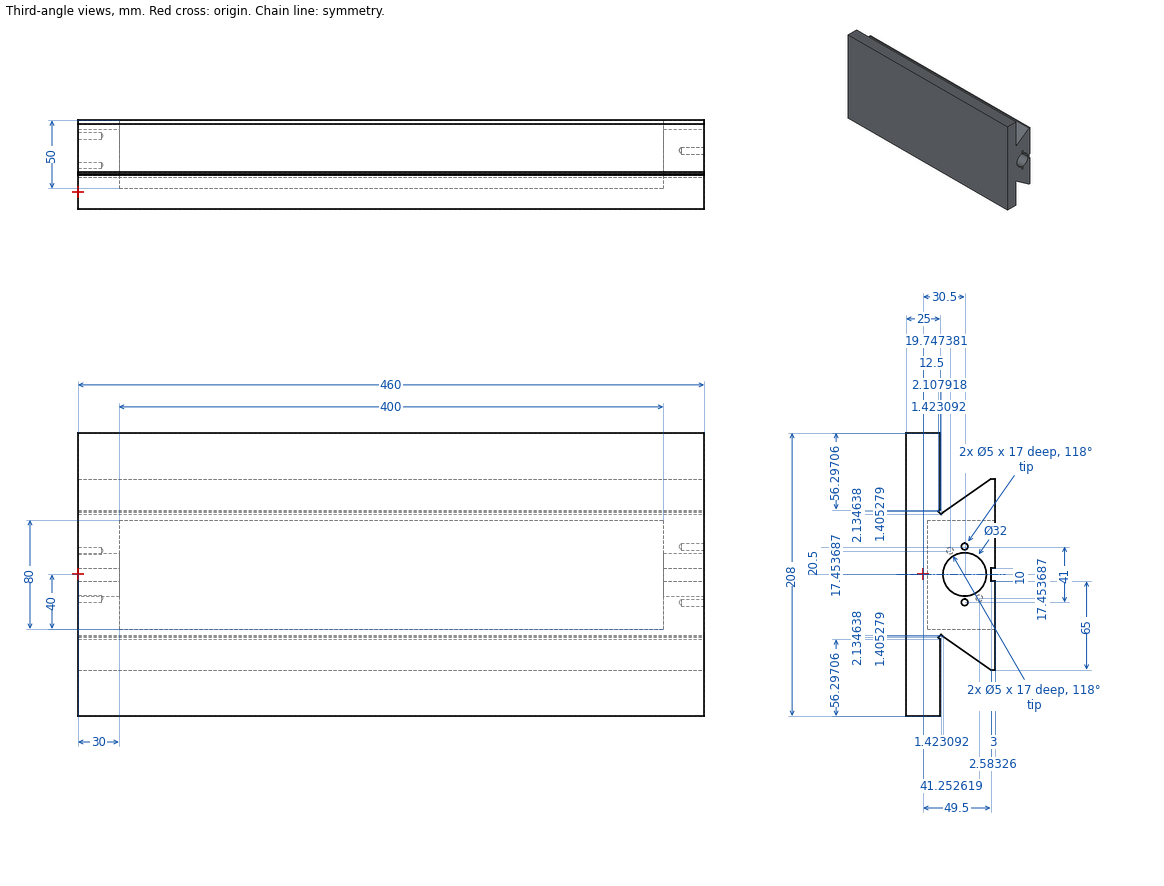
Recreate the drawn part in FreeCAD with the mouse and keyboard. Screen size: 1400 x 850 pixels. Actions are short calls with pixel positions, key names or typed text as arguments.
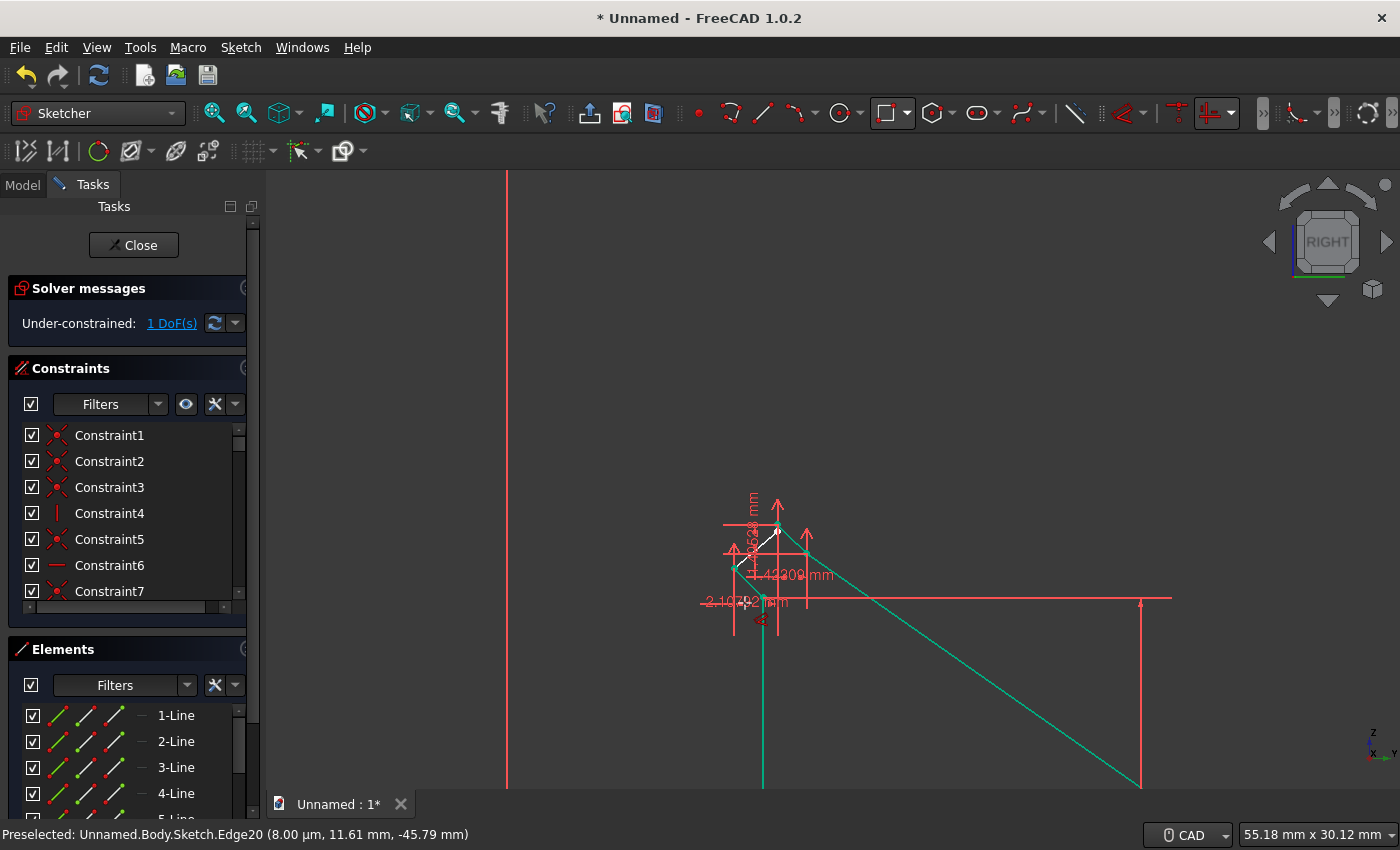
click(747, 558)
click(700, 559)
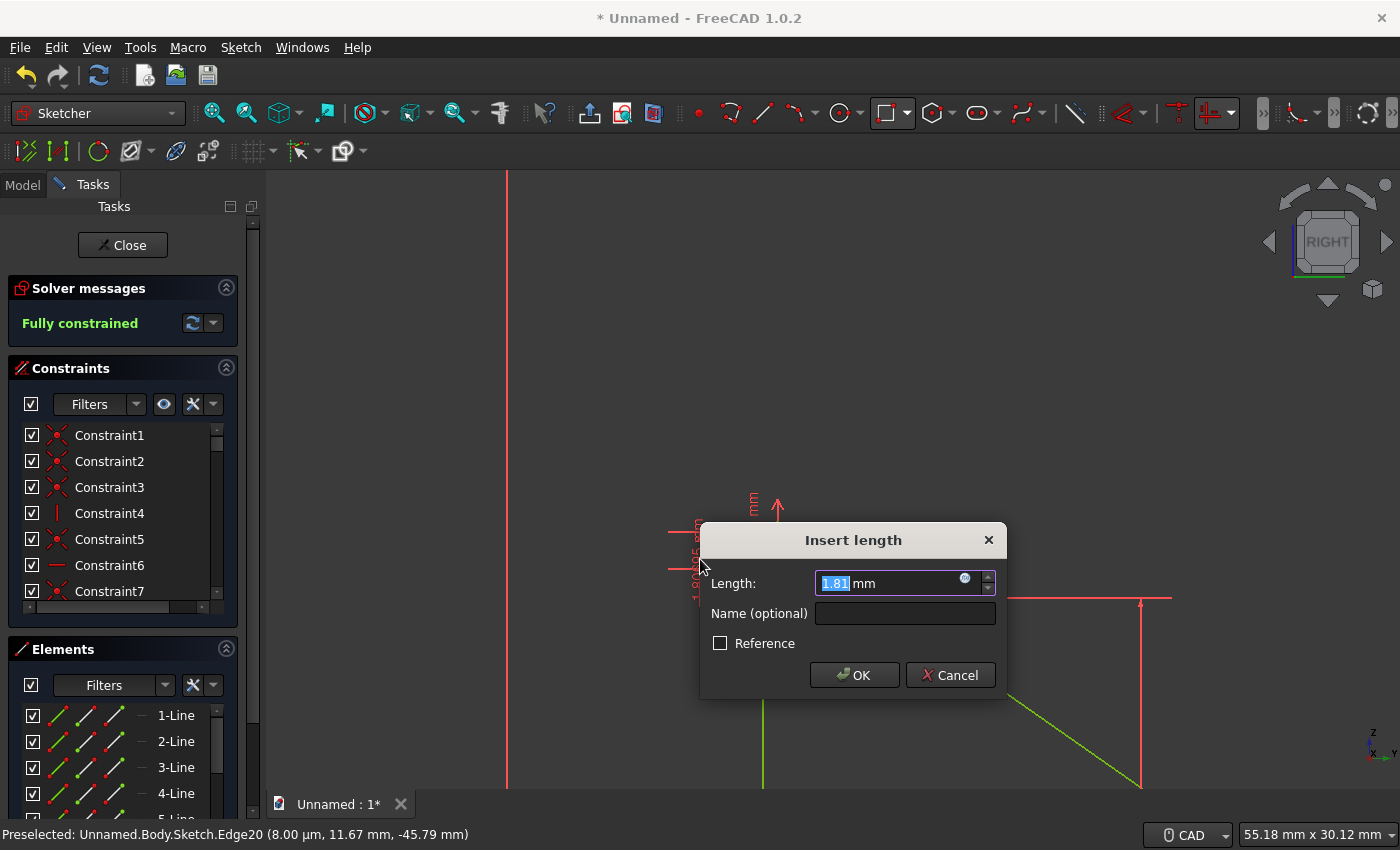
text(2.134638)
key(Return)
key(Escape)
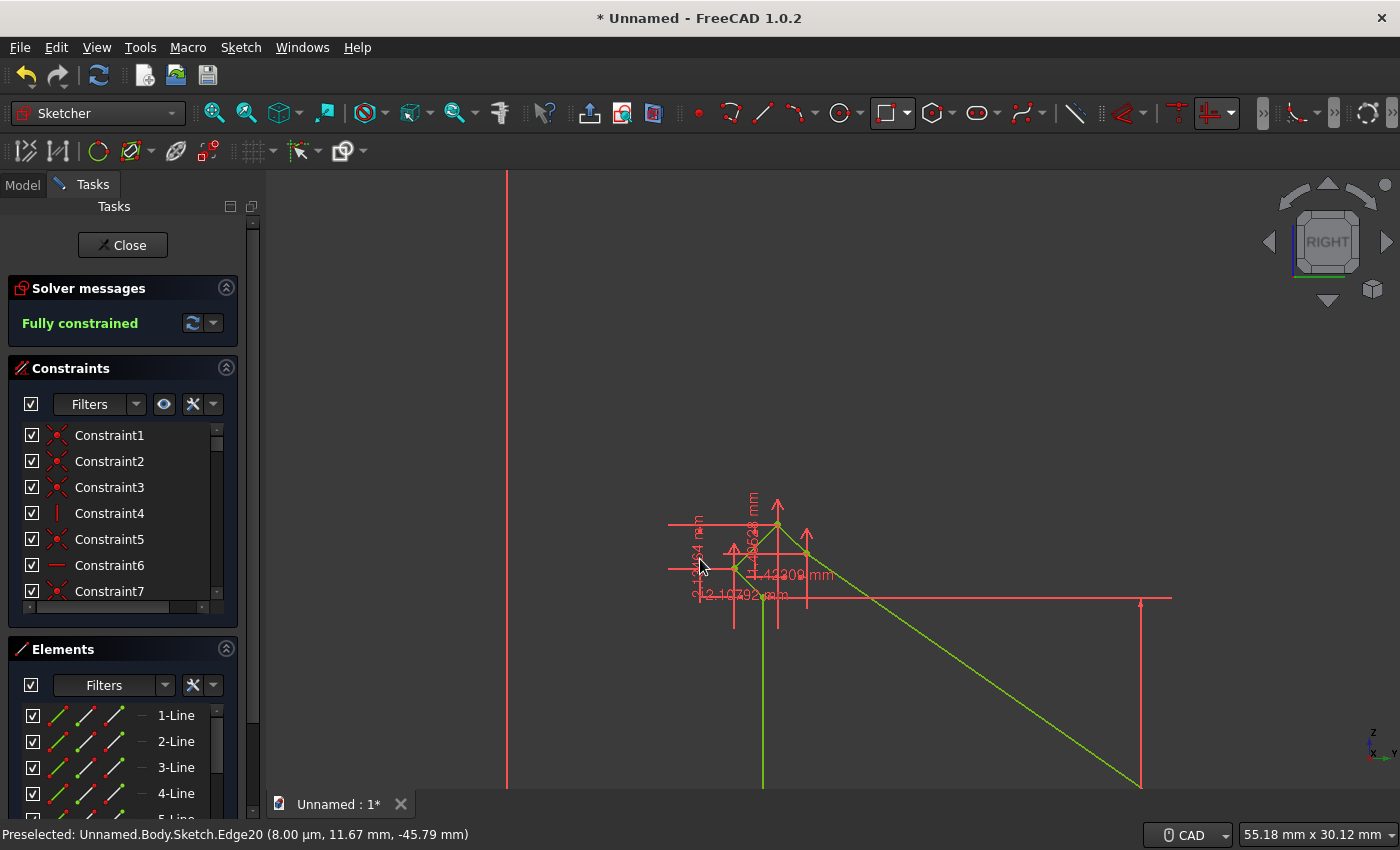
click(123, 245)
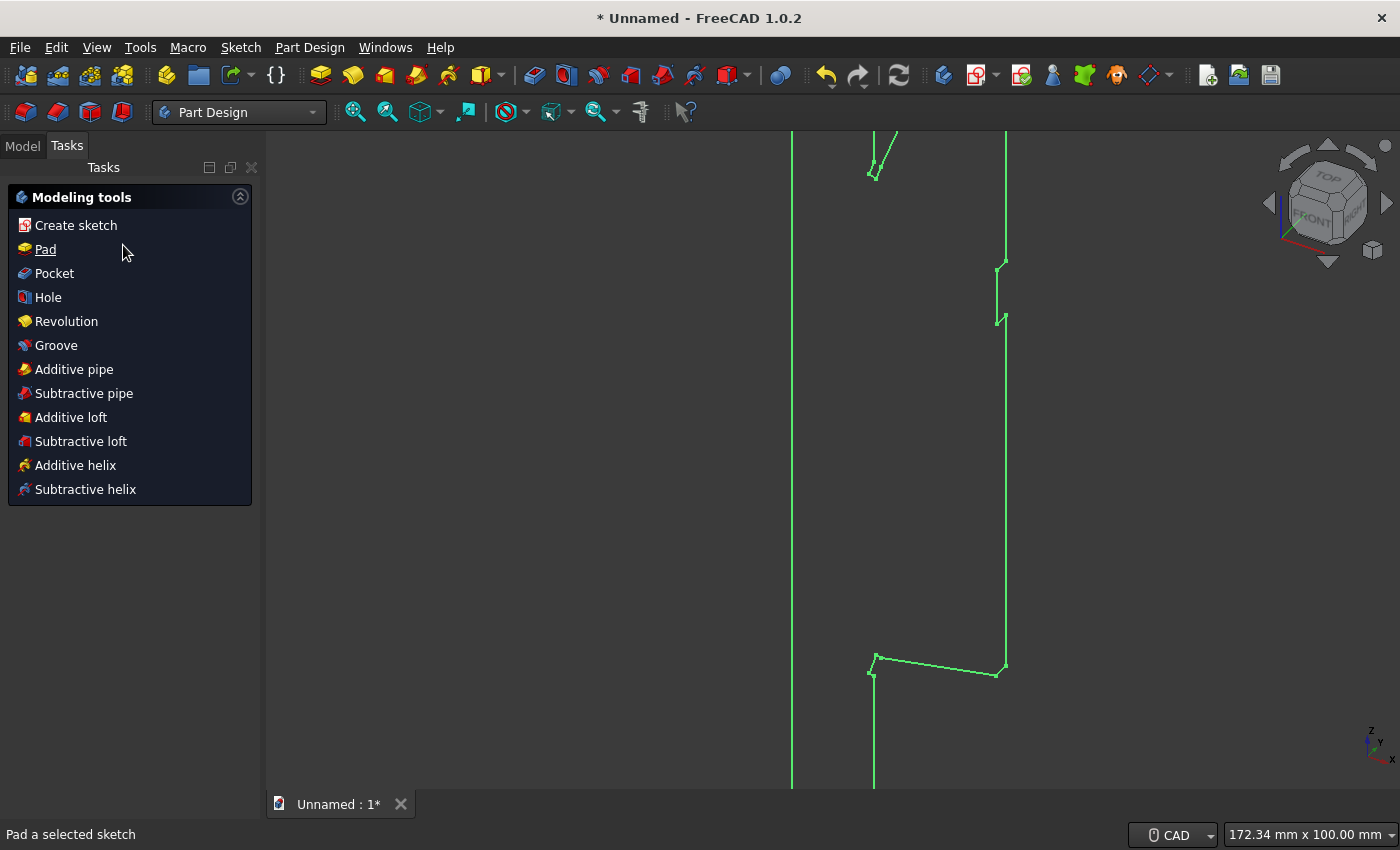
click(322, 76)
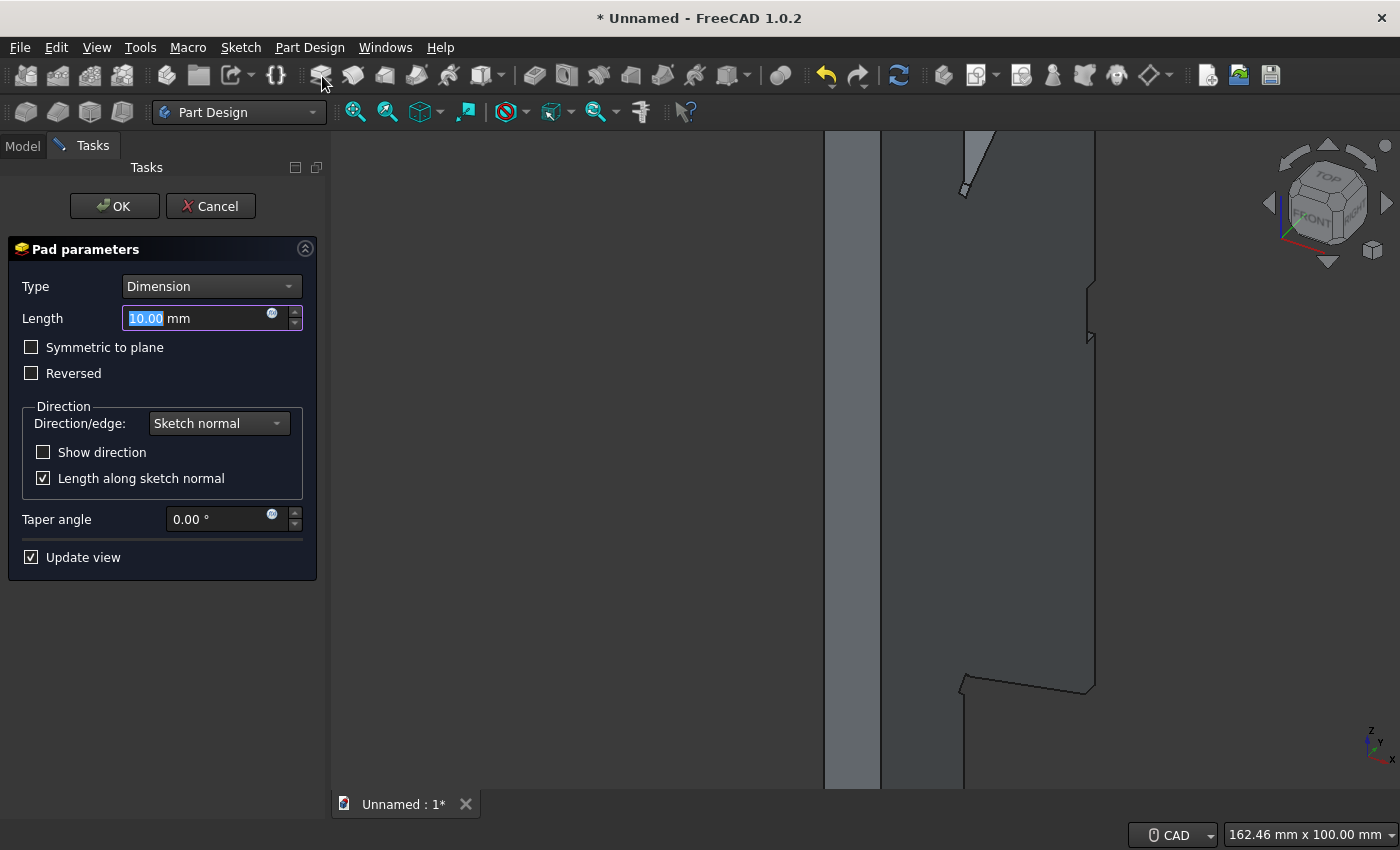
text(460)
key(Tab)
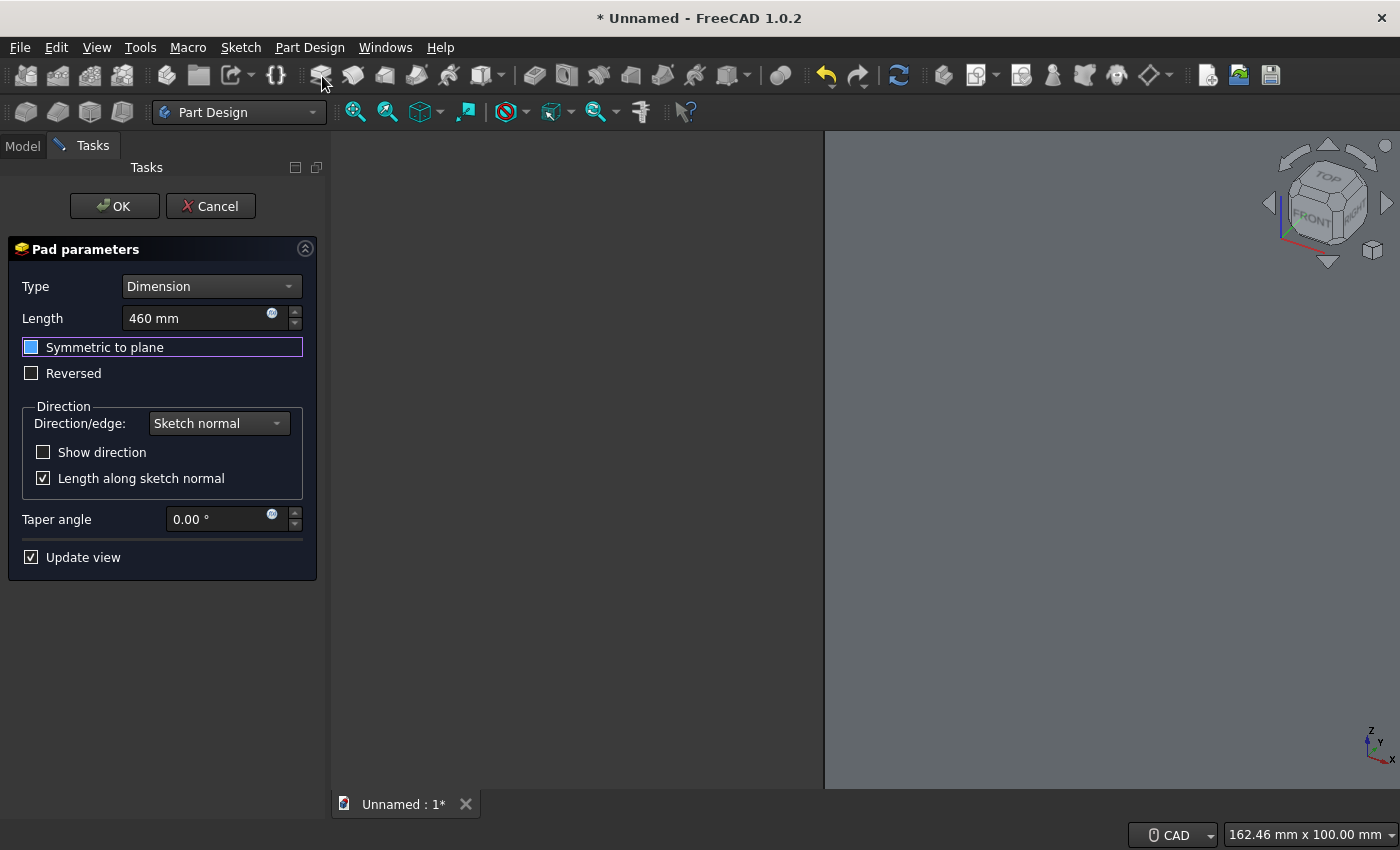
click(115, 206)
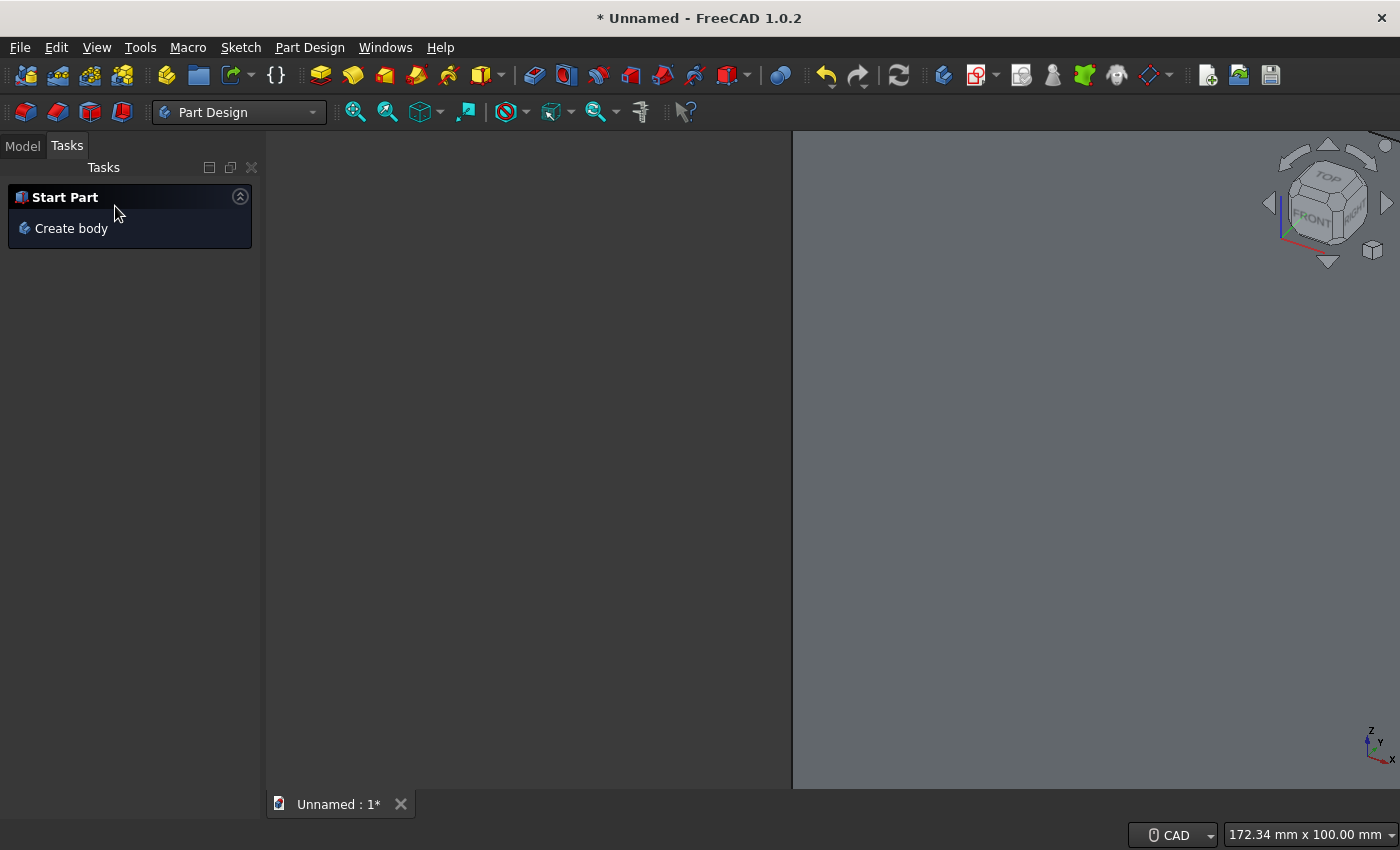
click(356, 112)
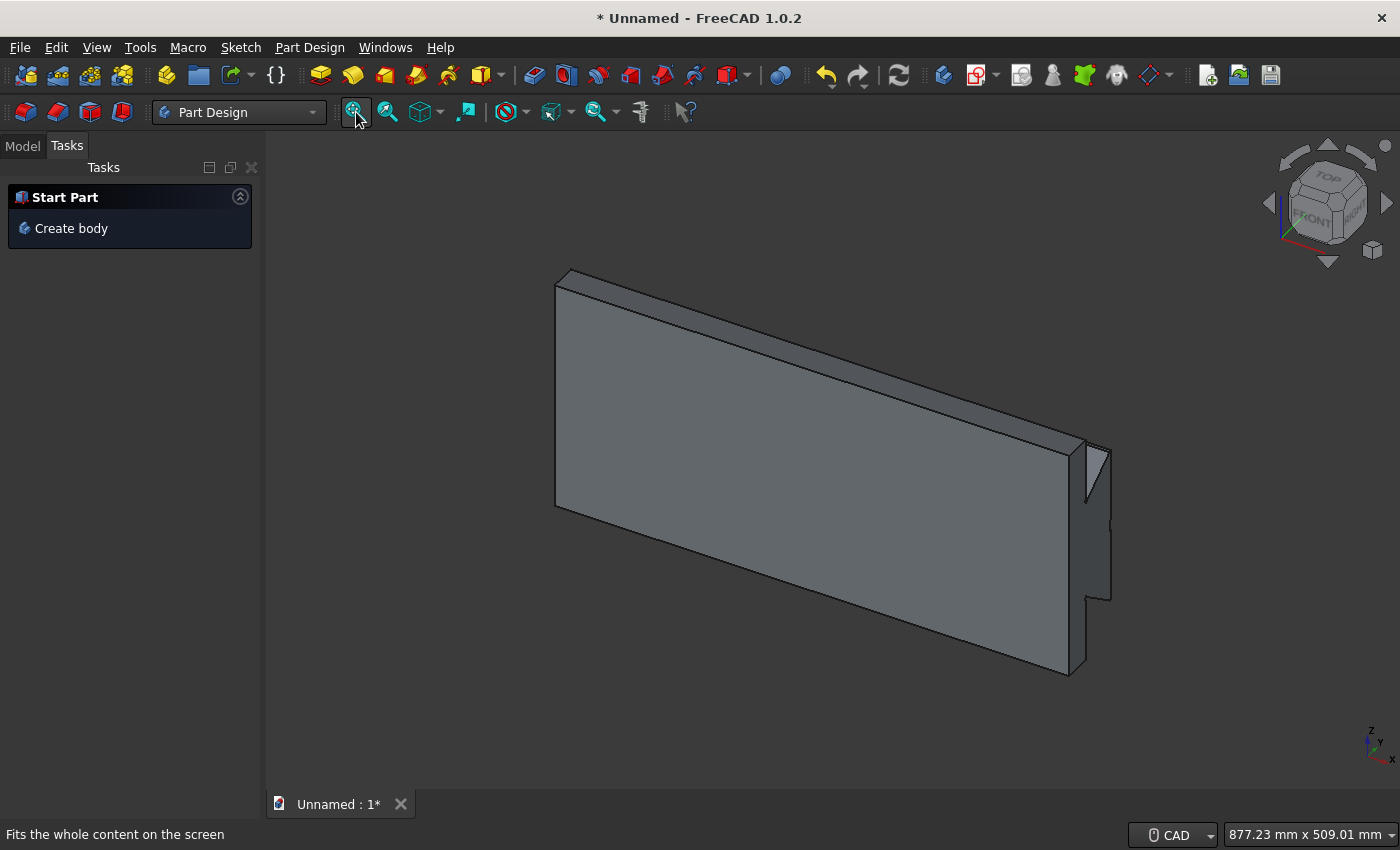
key(4)